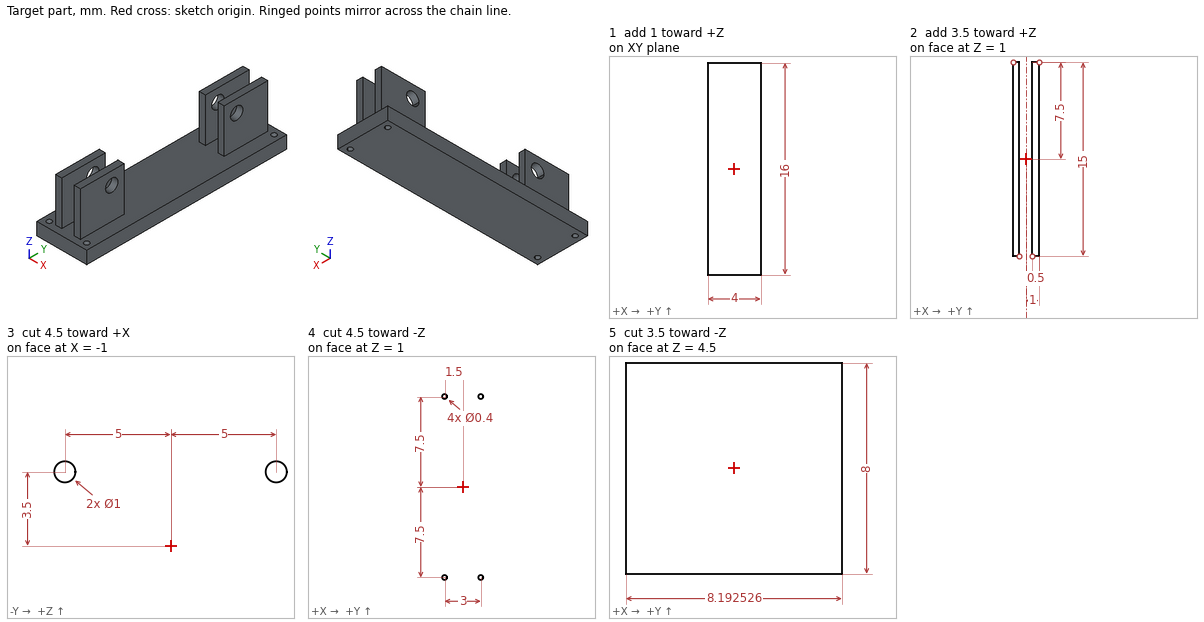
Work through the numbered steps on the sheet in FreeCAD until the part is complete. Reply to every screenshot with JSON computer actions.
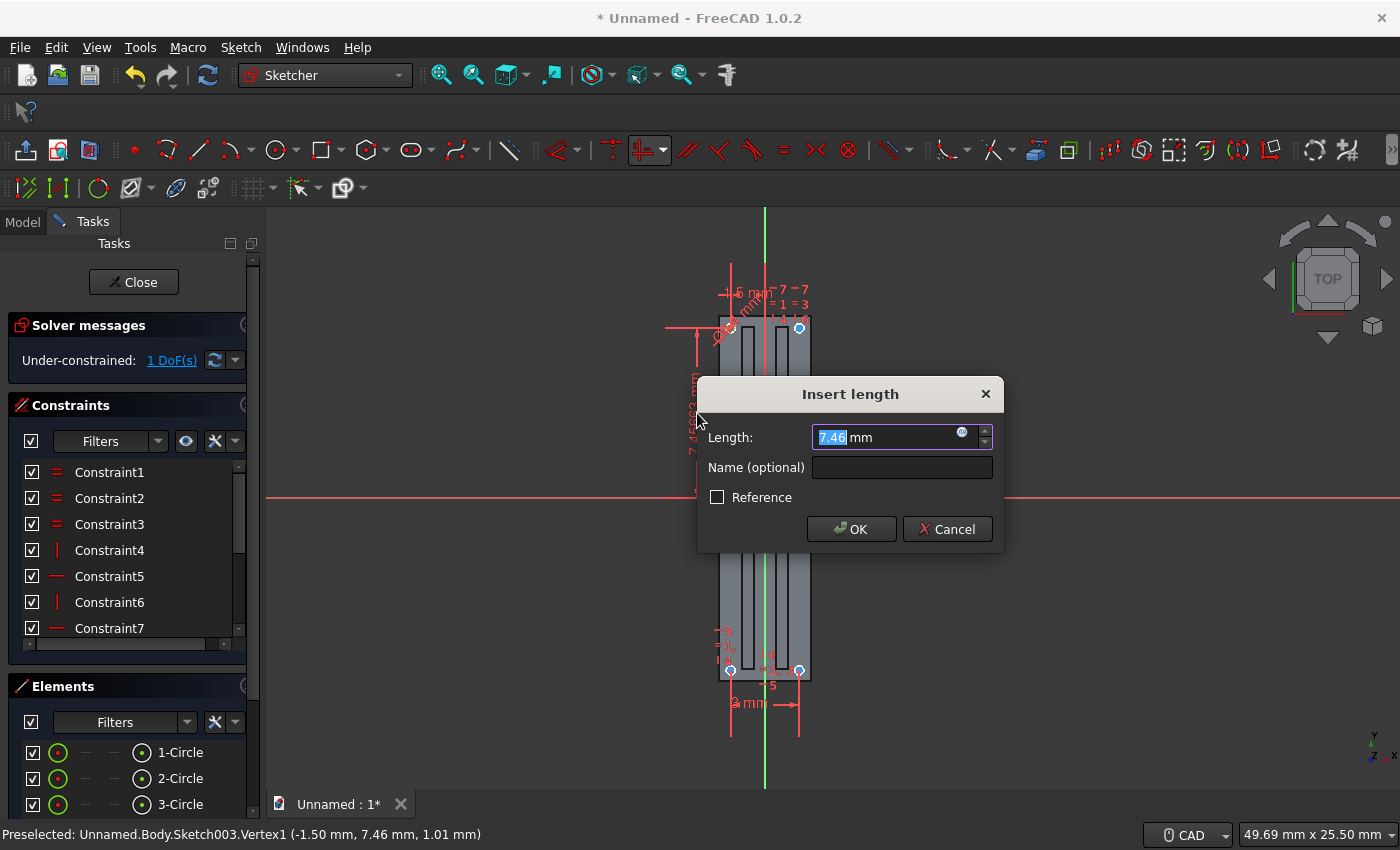
{"action": "type", "text": "7.5"}
{"action": "key", "text": "Return"}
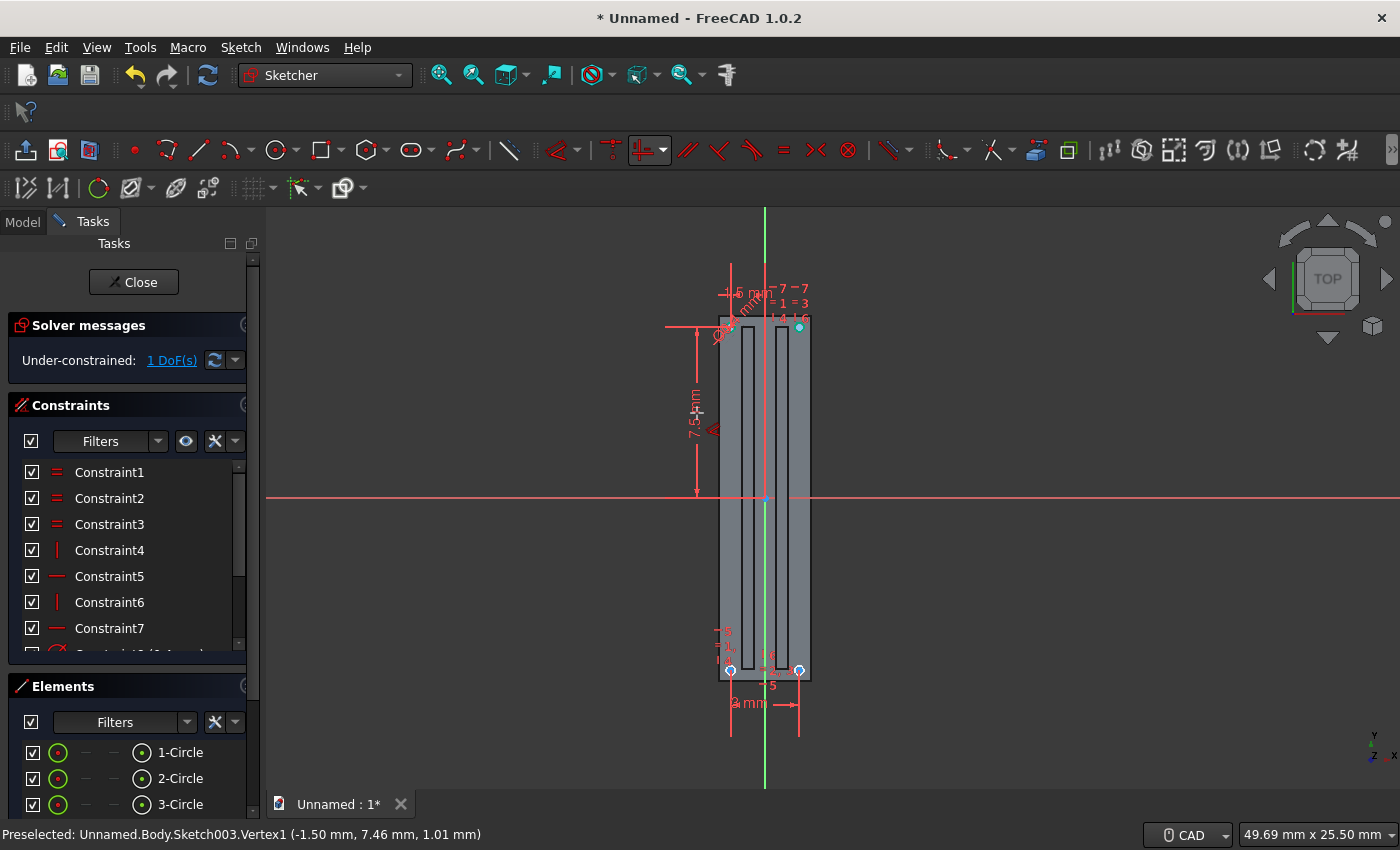
{"action": "left_click", "coordinate": [731, 670]}
{"action": "left_click", "coordinate": [697, 584]}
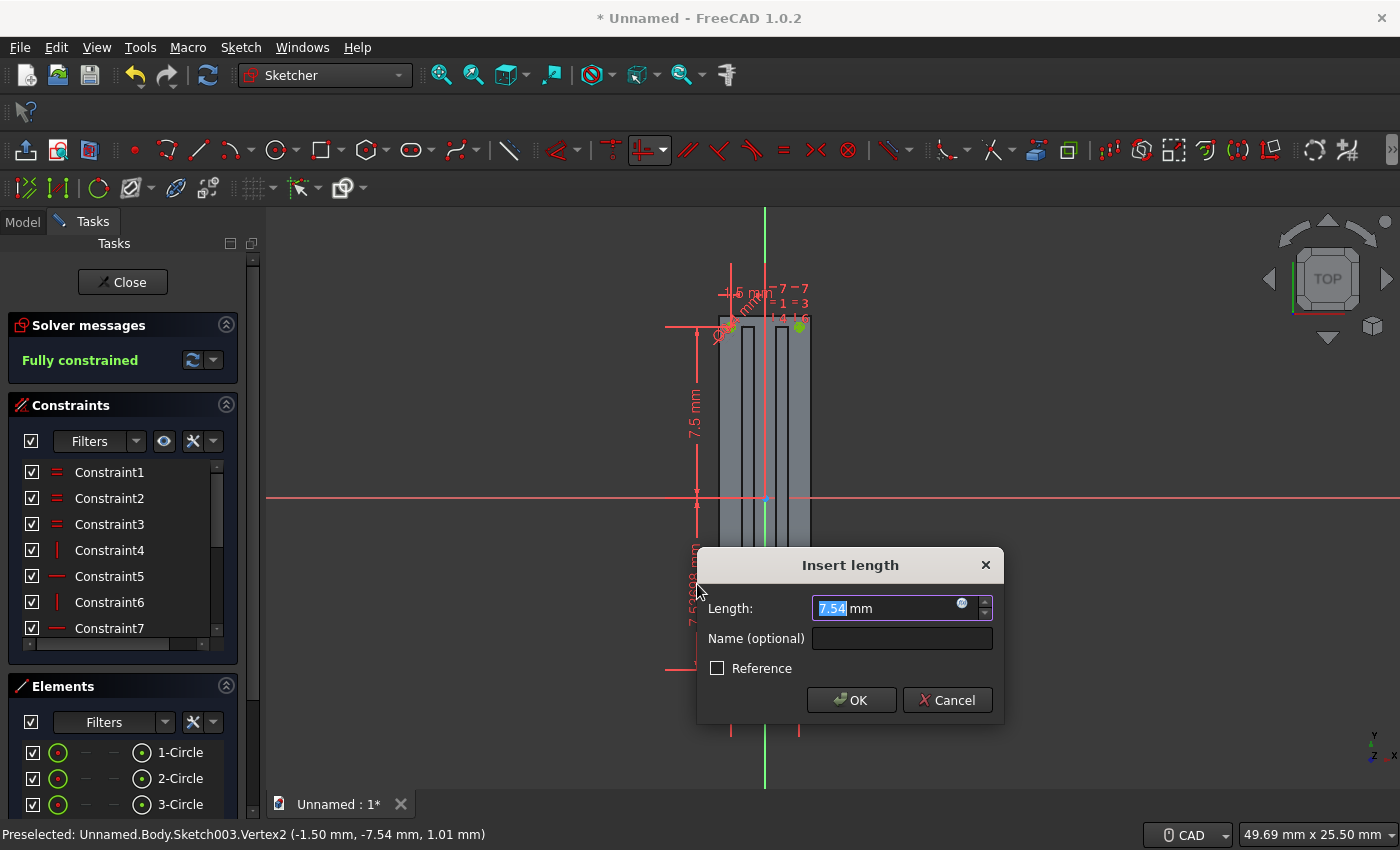
{"action": "type", "text": "7.5"}
{"action": "key", "text": "Return"}
{"action": "key", "text": "Escape"}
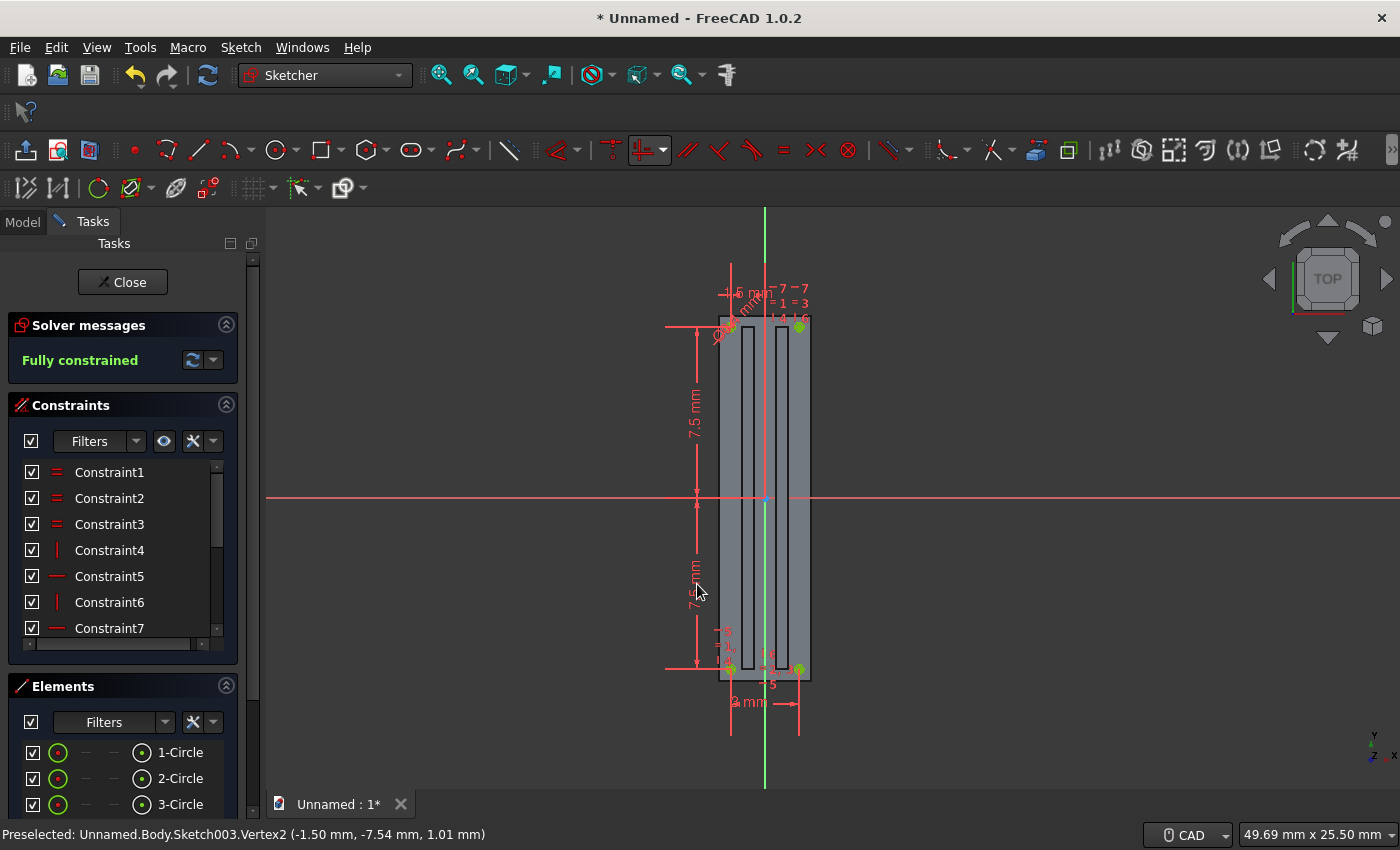
{"action": "left_click", "coordinate": [123, 282]}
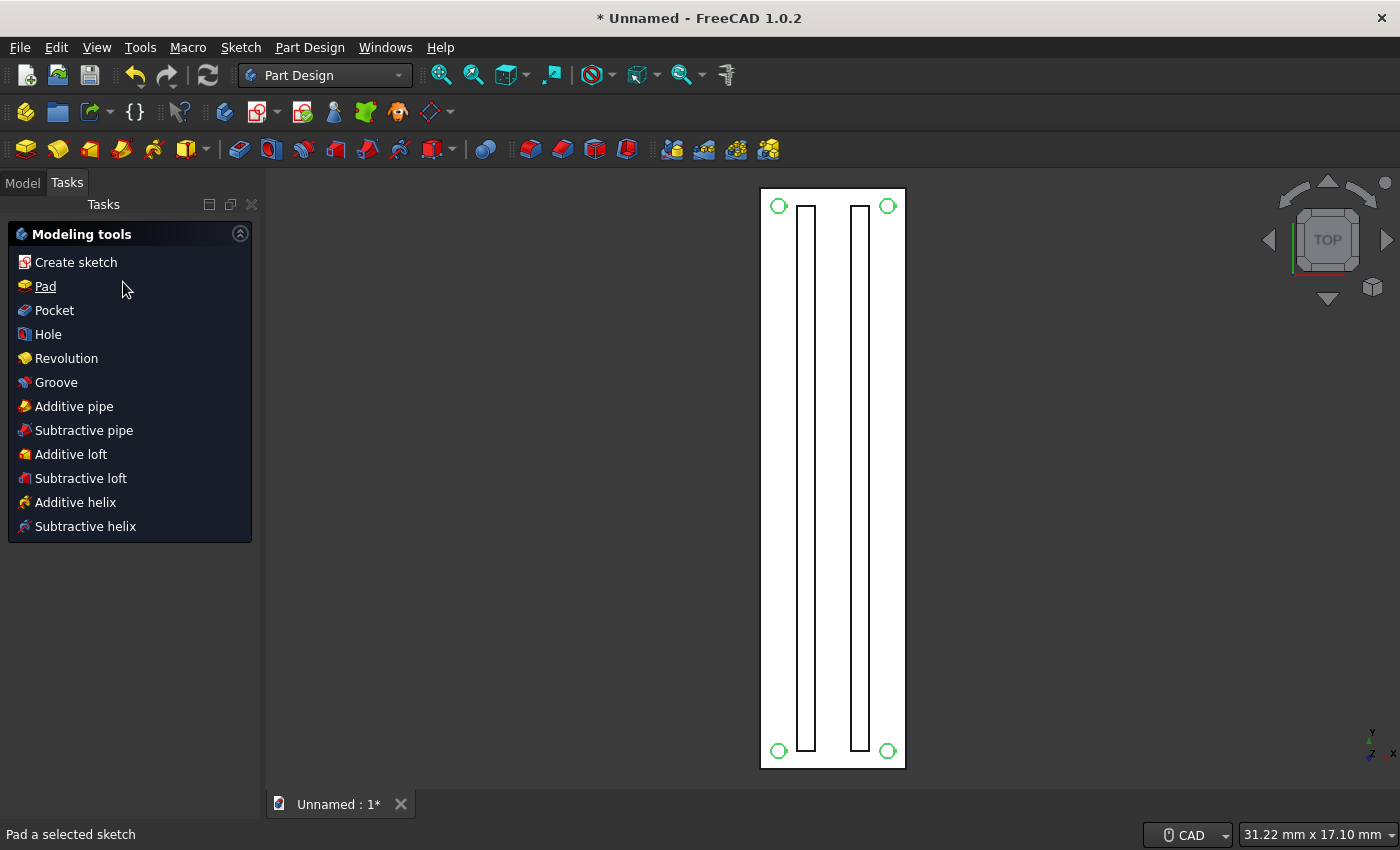
{"action": "left_click", "coordinate": [240, 150]}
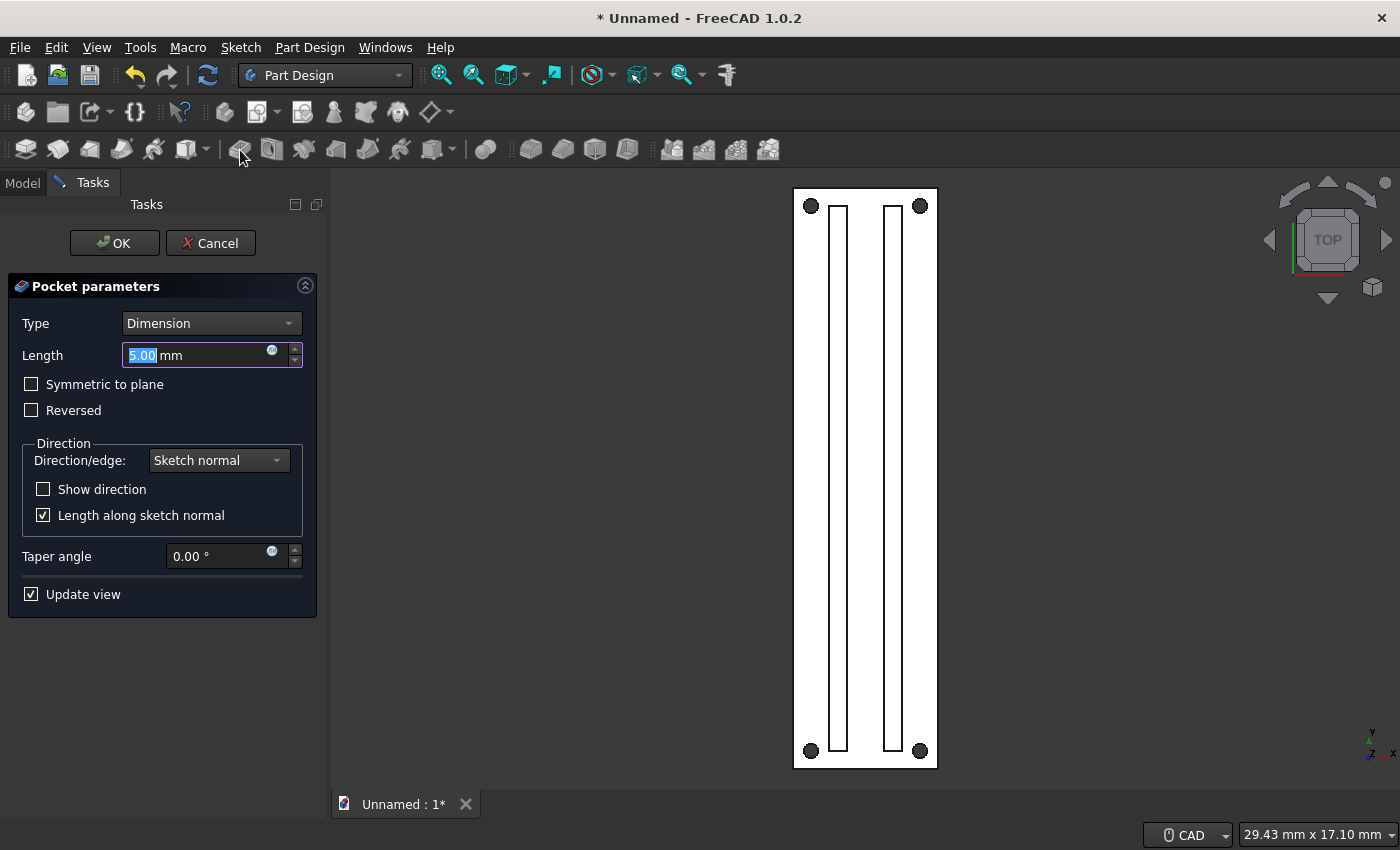
{"action": "type", "text": "4.5"}
{"action": "key", "text": "Tab"}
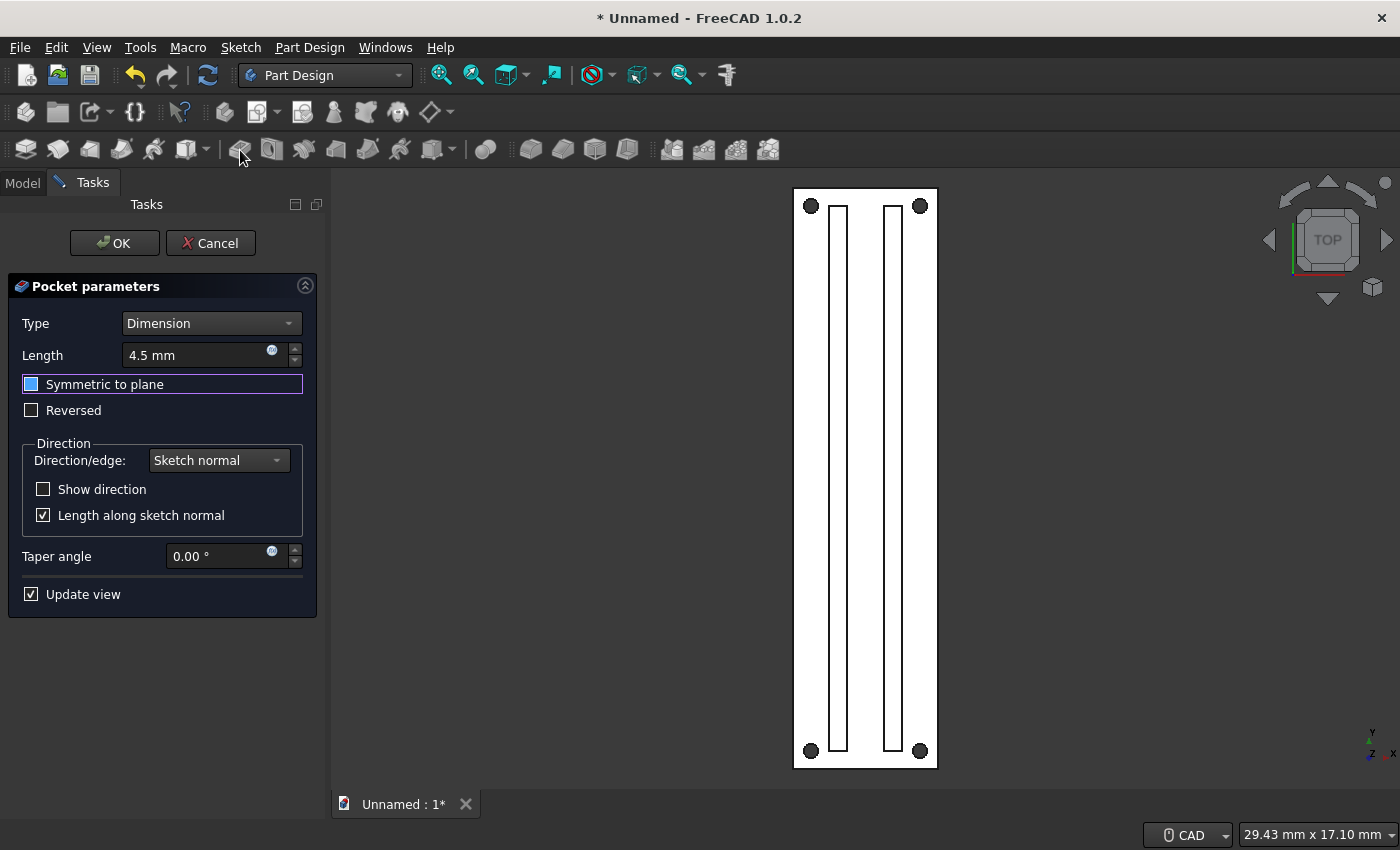
{"action": "left_click", "coordinate": [115, 243]}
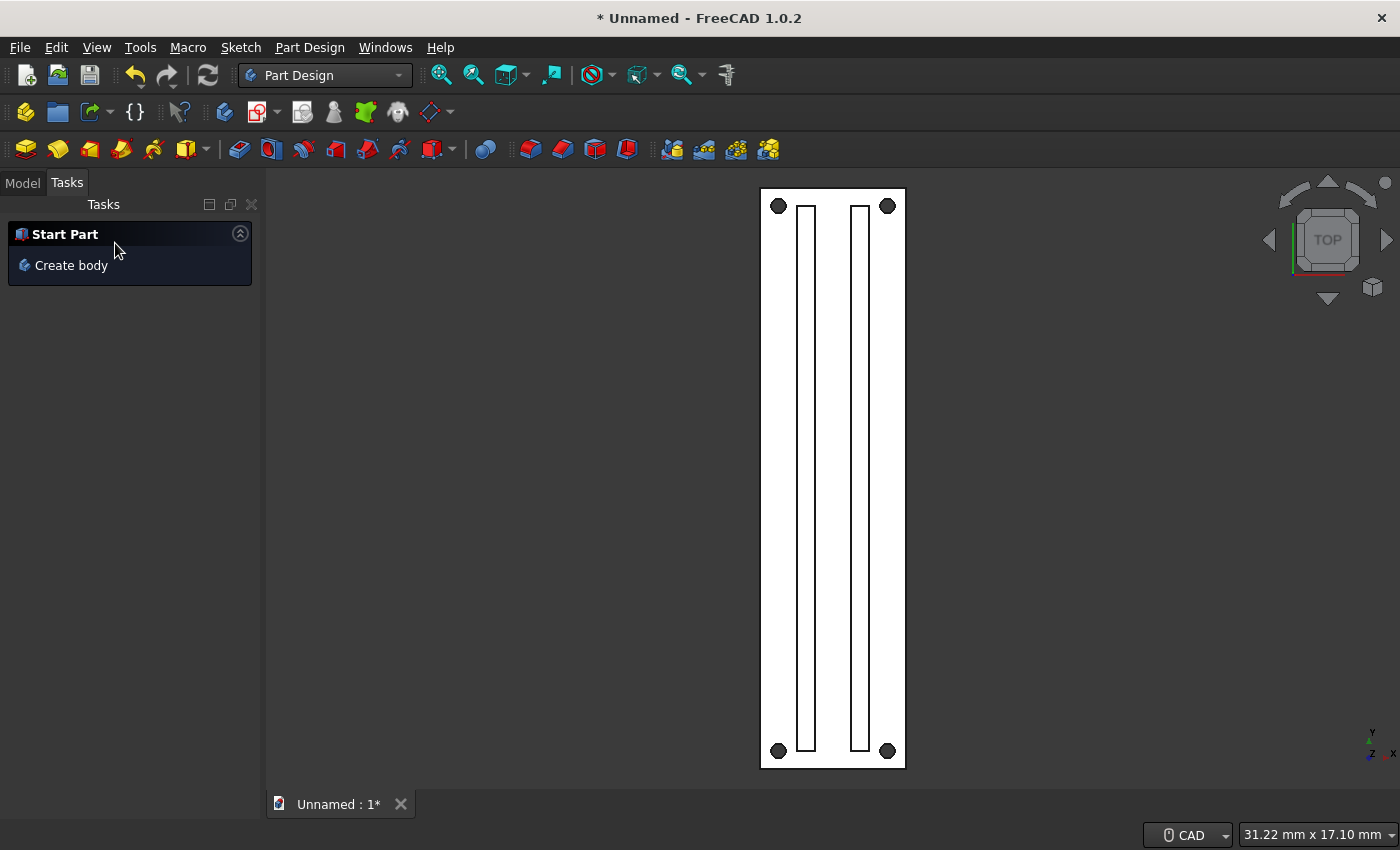
{"action": "left_click", "coordinate": [860, 244]}